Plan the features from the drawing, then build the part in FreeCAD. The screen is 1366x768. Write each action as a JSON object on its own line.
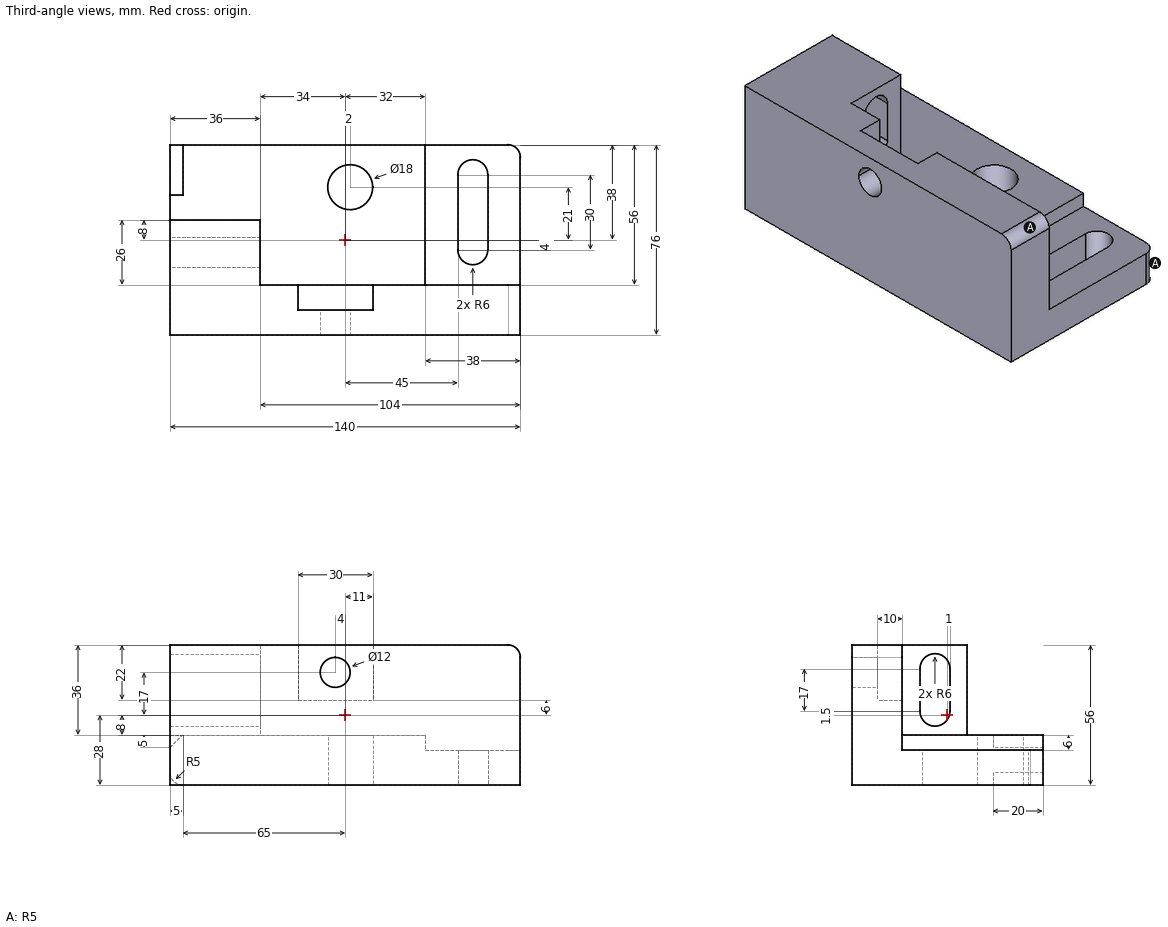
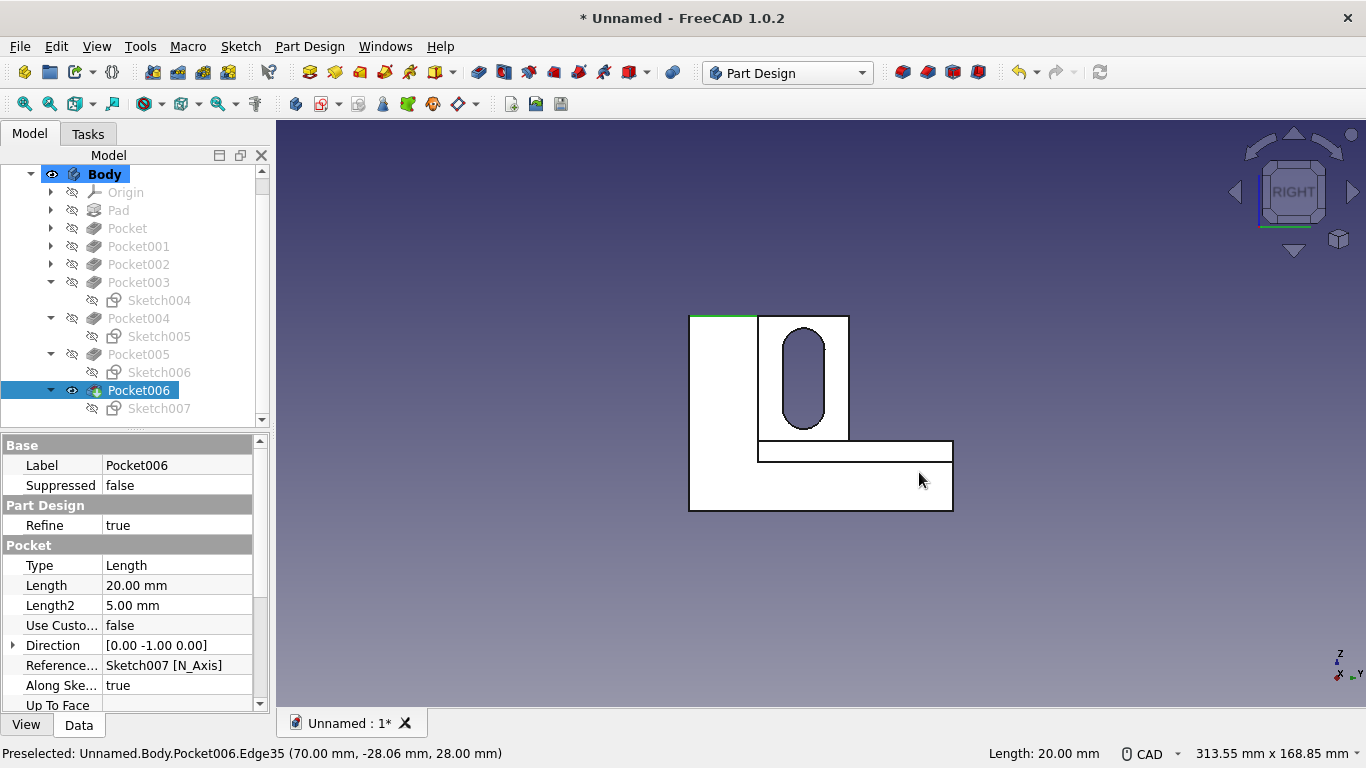
{"action": "left_click", "coordinate": [25, 104]}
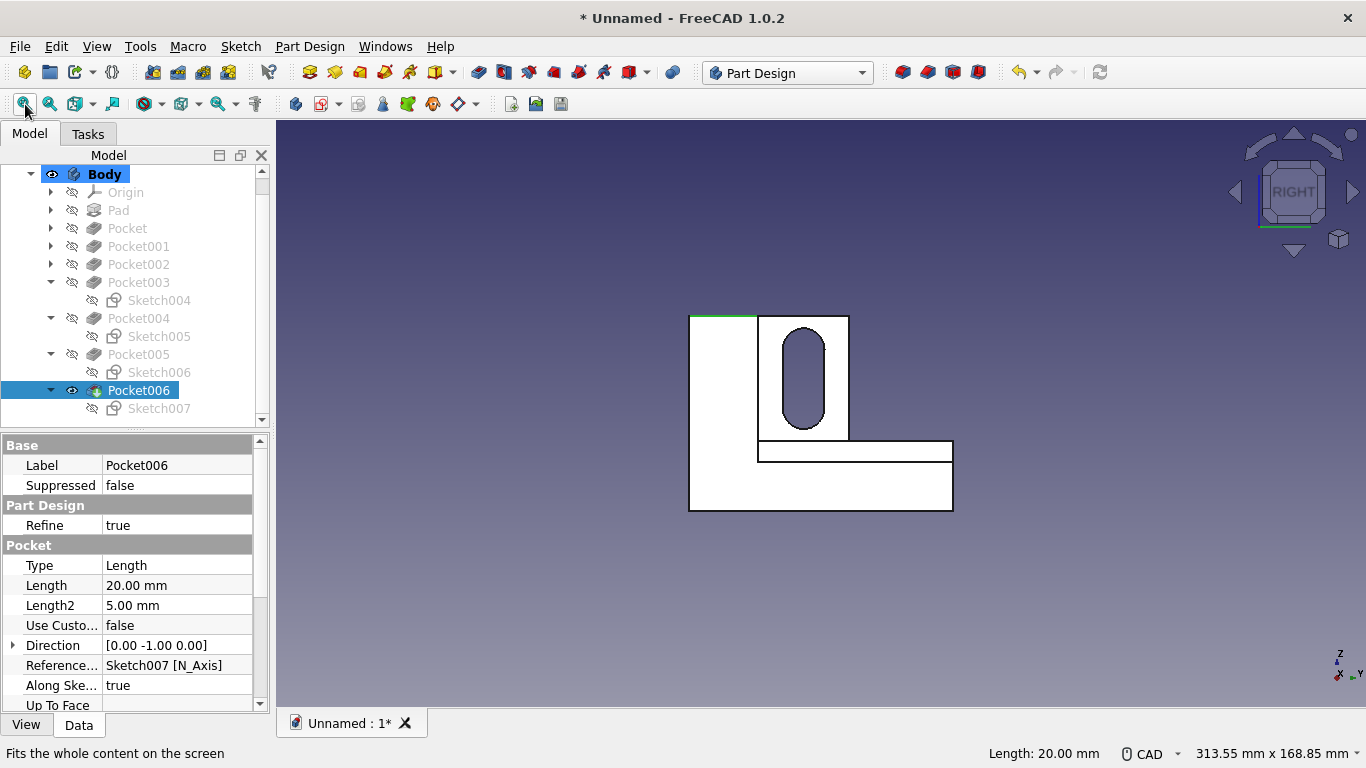
{"action": "left_click", "coordinate": [953, 486], "text": "ctrl"}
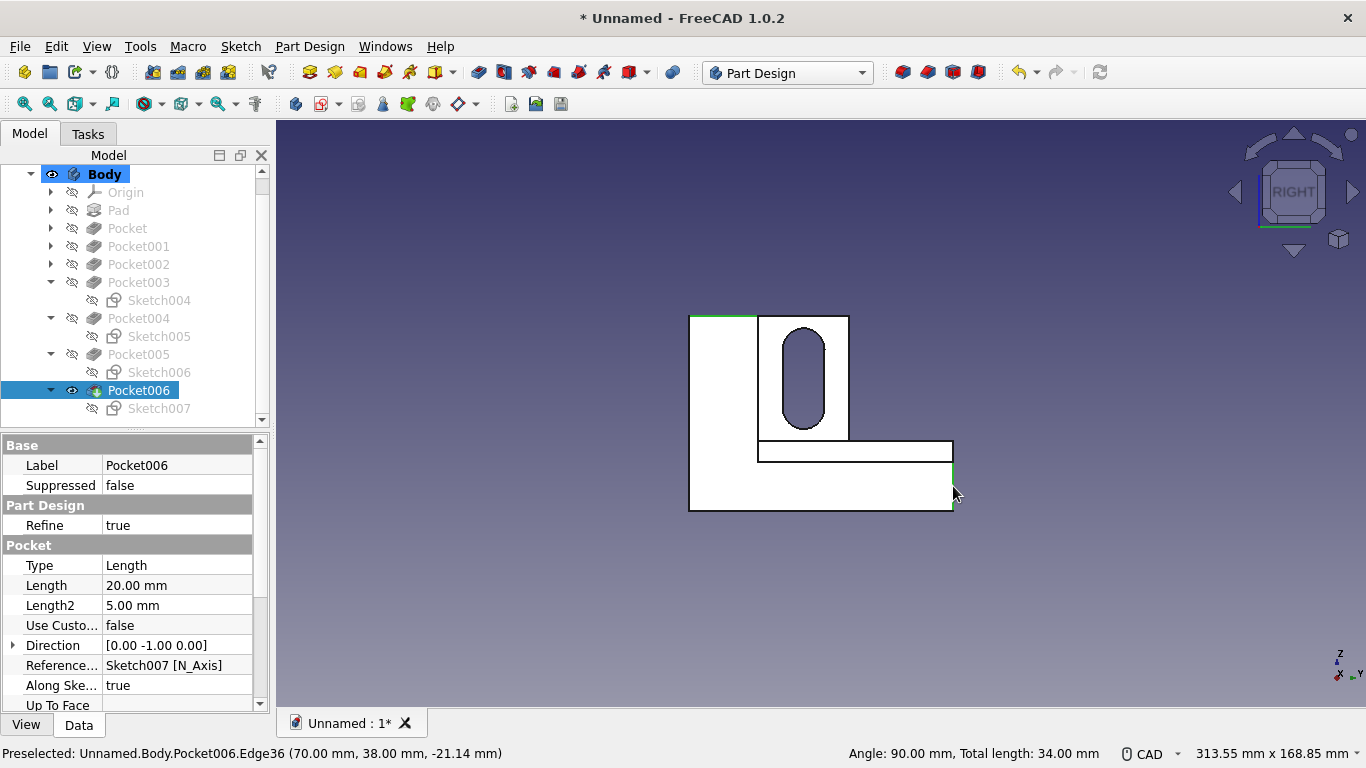
{"action": "left_click", "coordinate": [903, 72]}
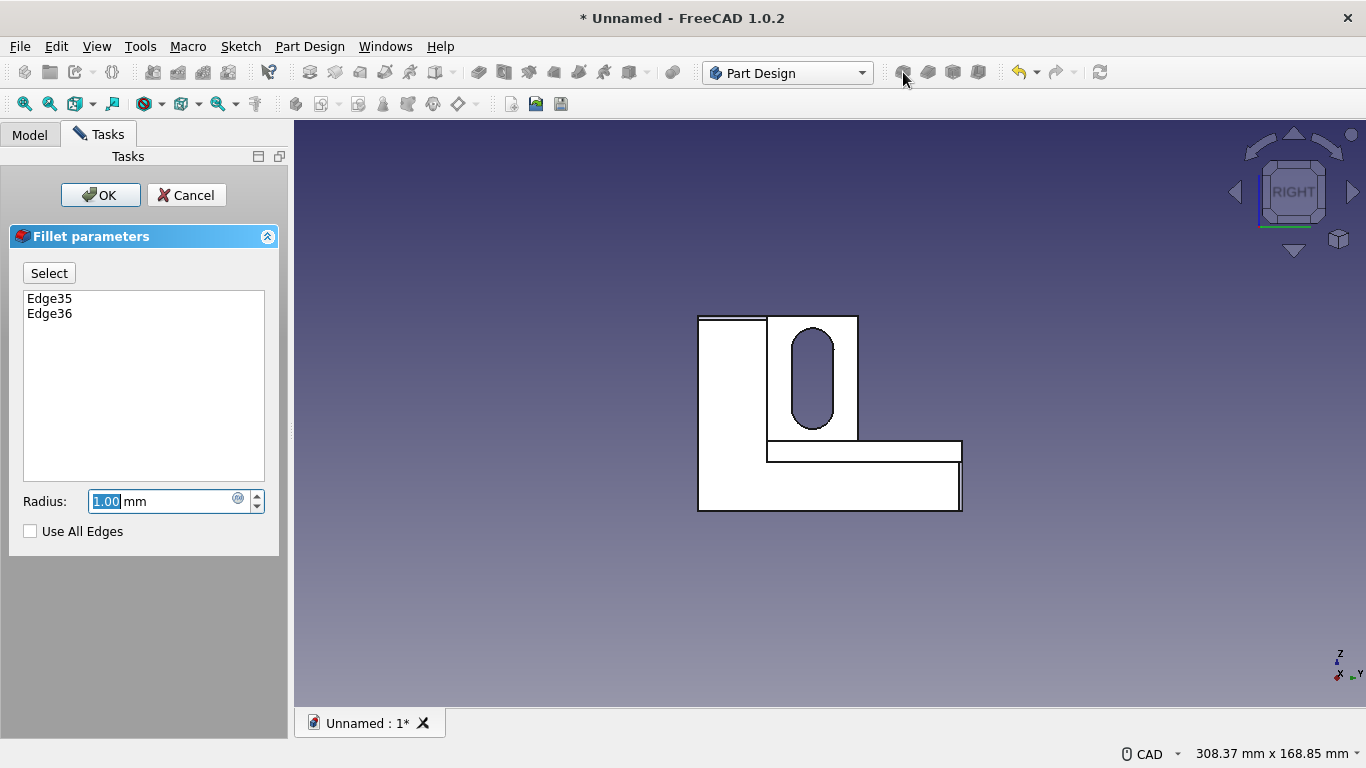
{"action": "type", "text": "5"}
{"action": "key", "text": "Tab"}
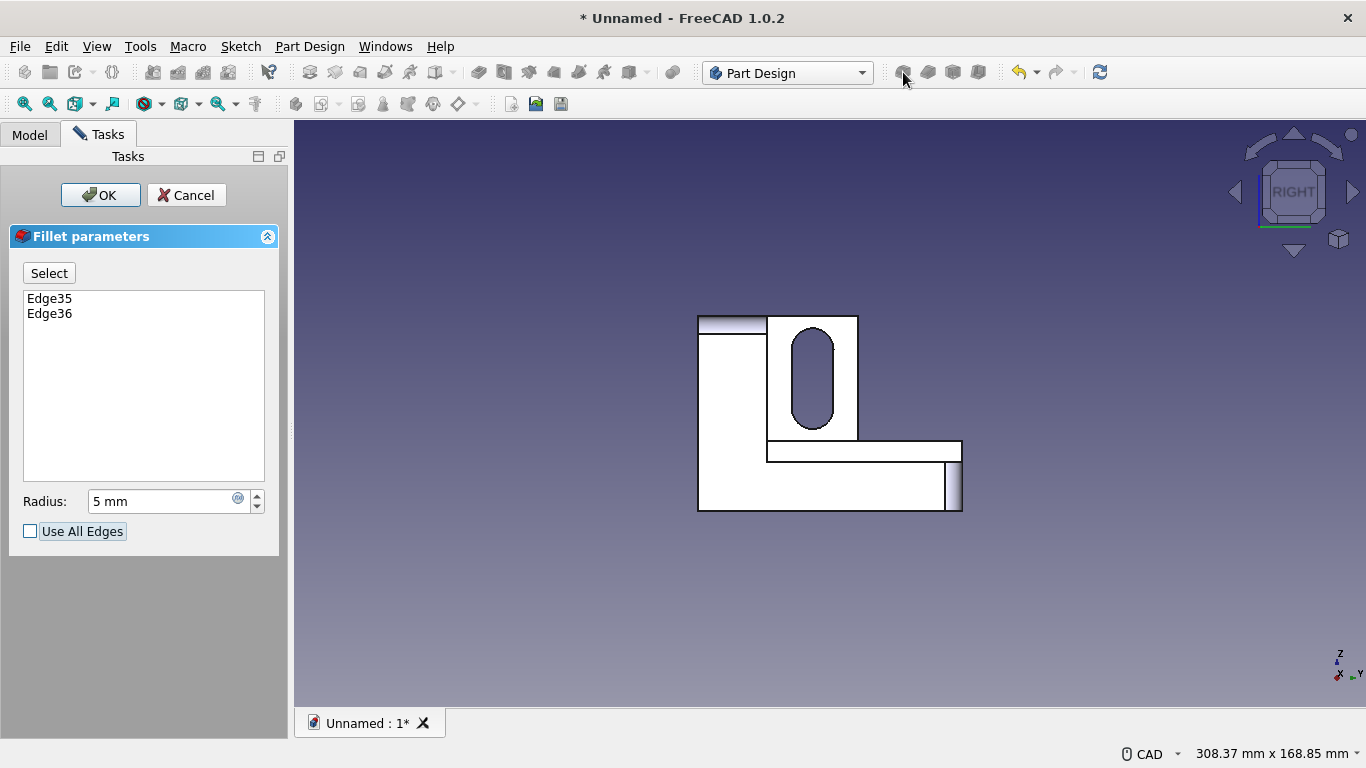
{"action": "left_click", "coordinate": [101, 195]}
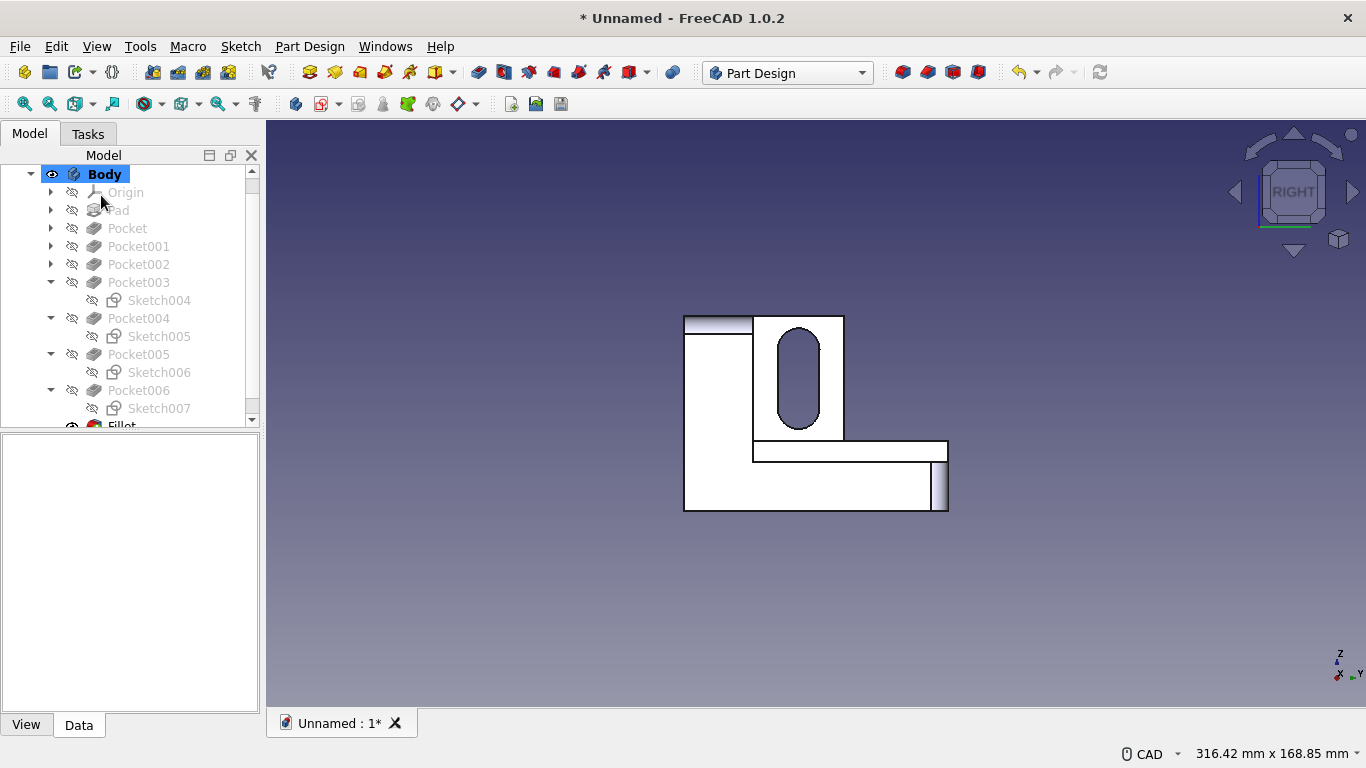
{"action": "key", "text": "0"}